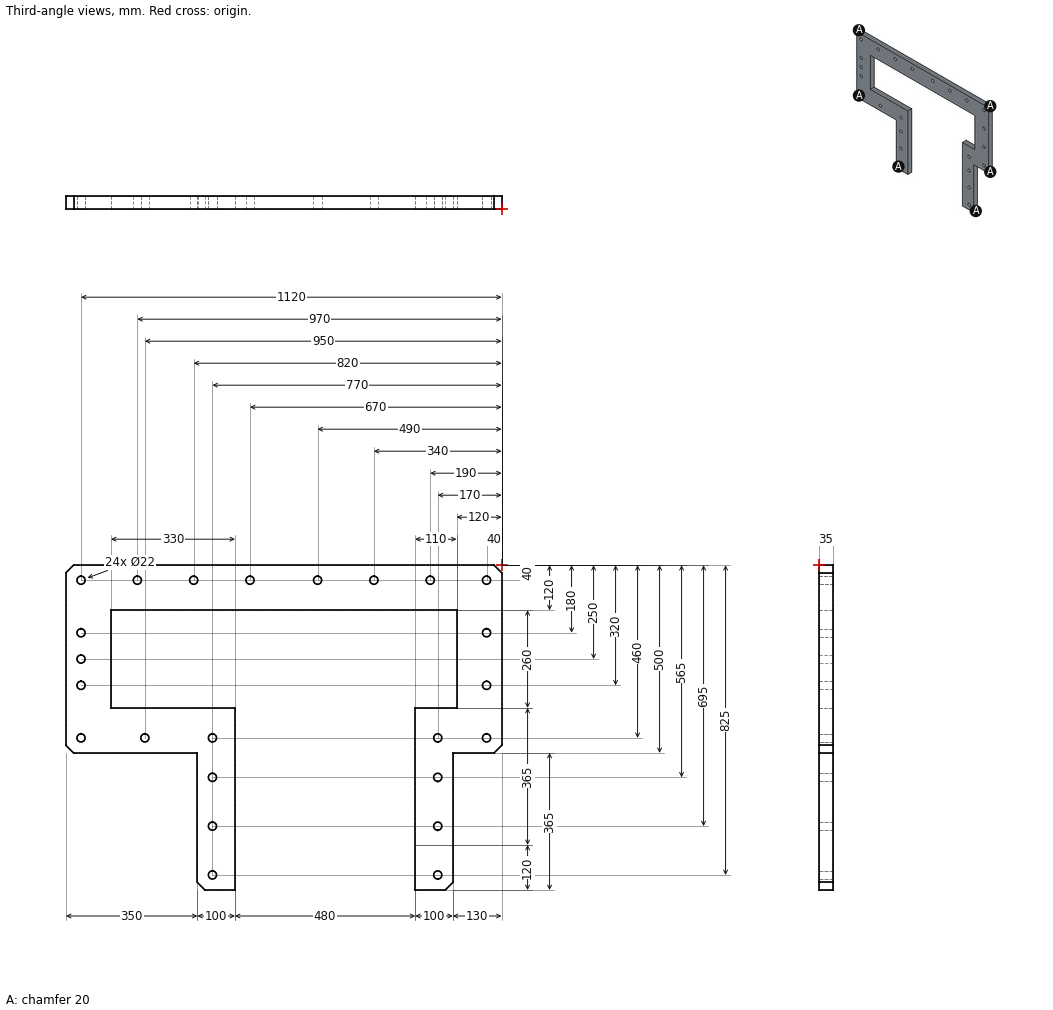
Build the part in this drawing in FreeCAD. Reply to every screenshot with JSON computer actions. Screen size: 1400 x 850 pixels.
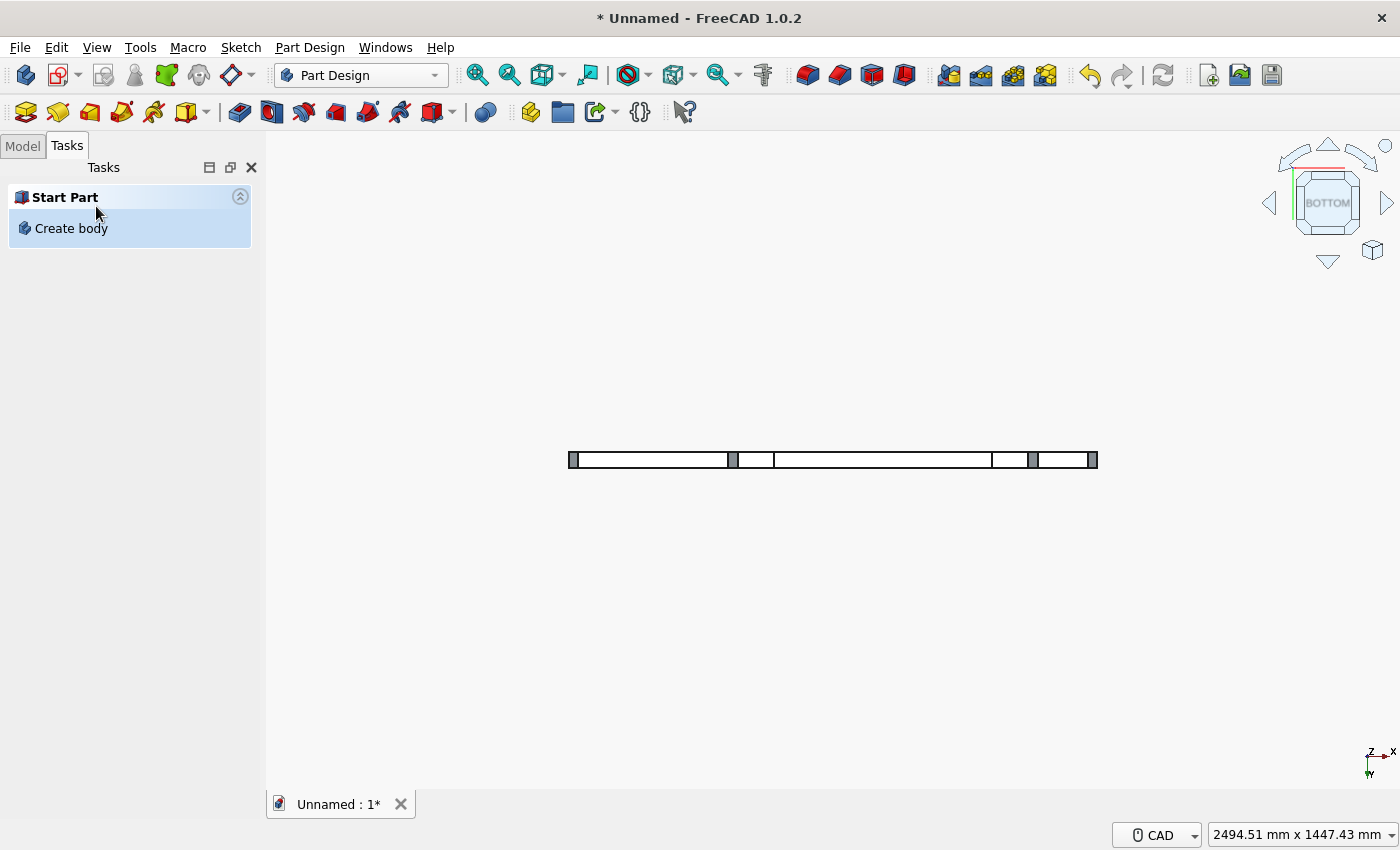
{"action": "key", "text": "4"}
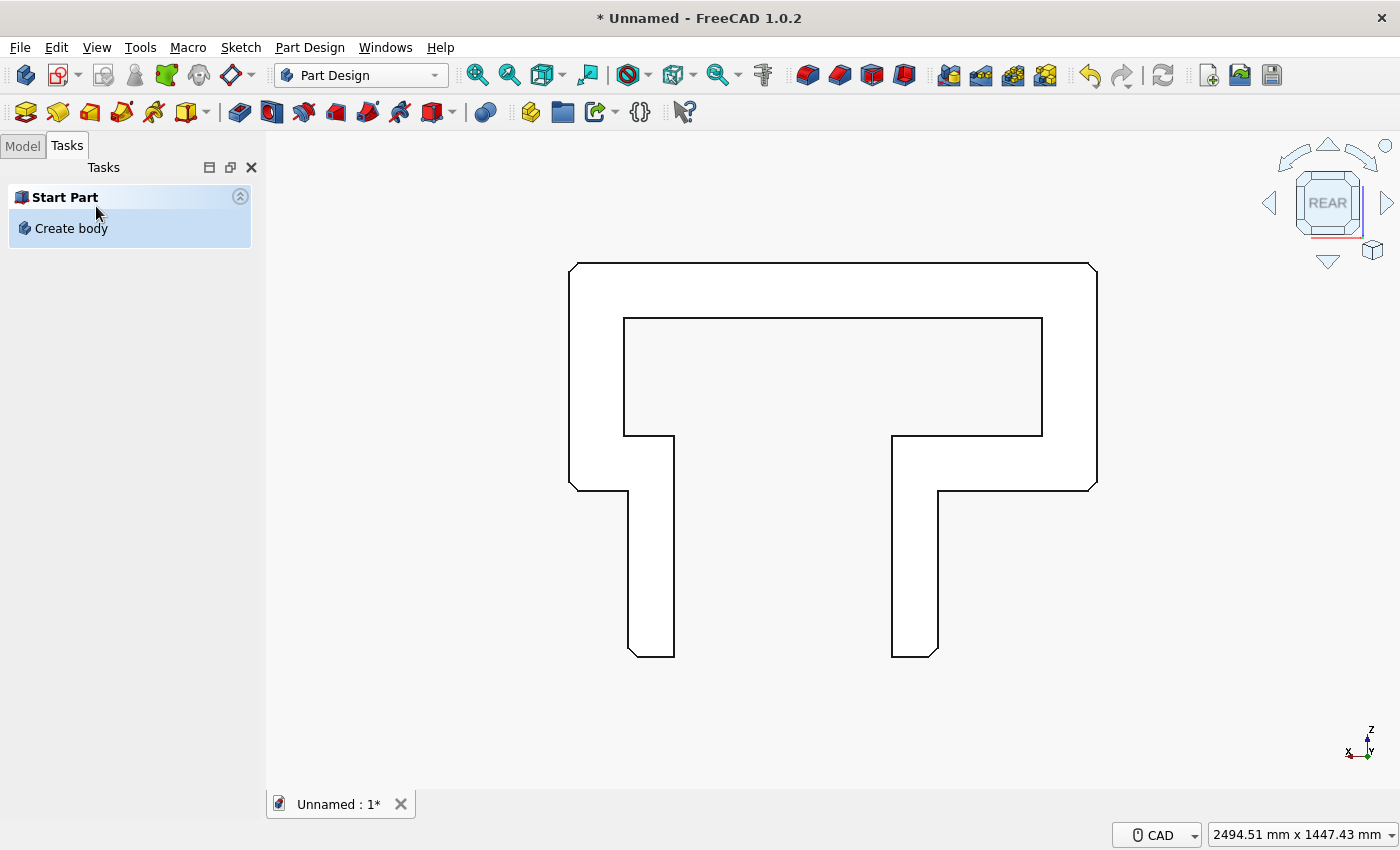
{"action": "left_click", "coordinate": [1059, 459]}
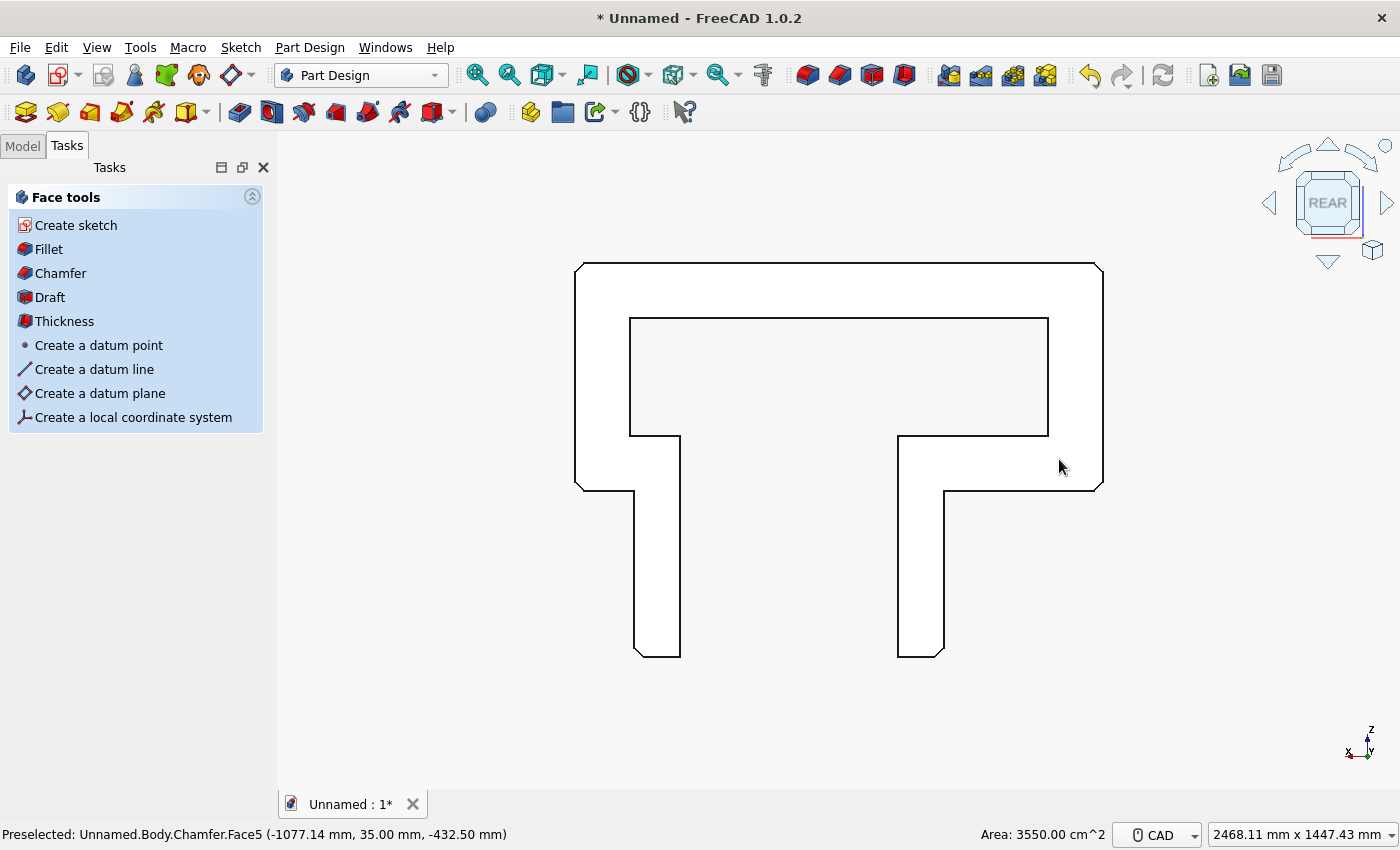
{"action": "left_click", "coordinate": [58, 76]}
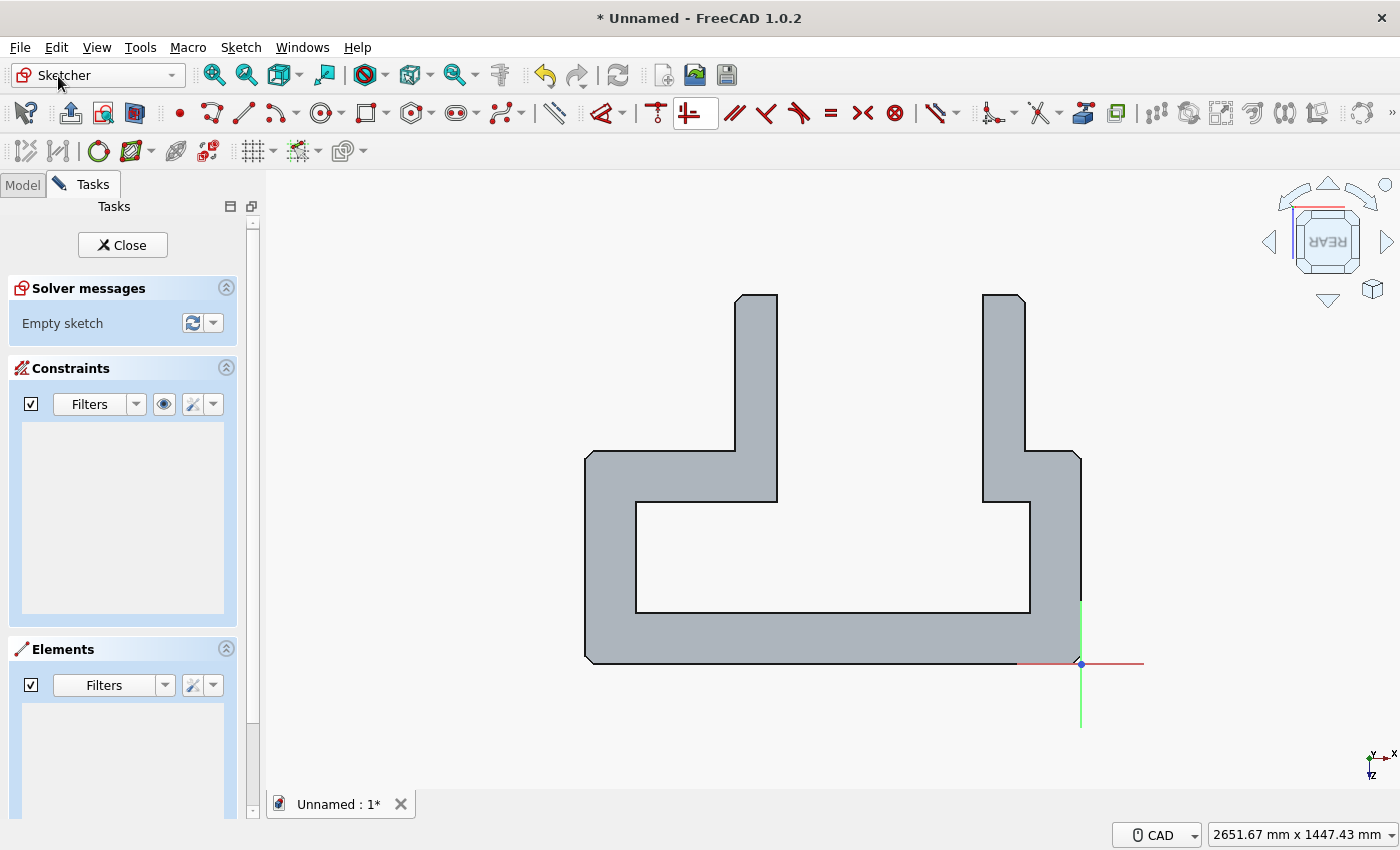
{"action": "key", "text": "g c"}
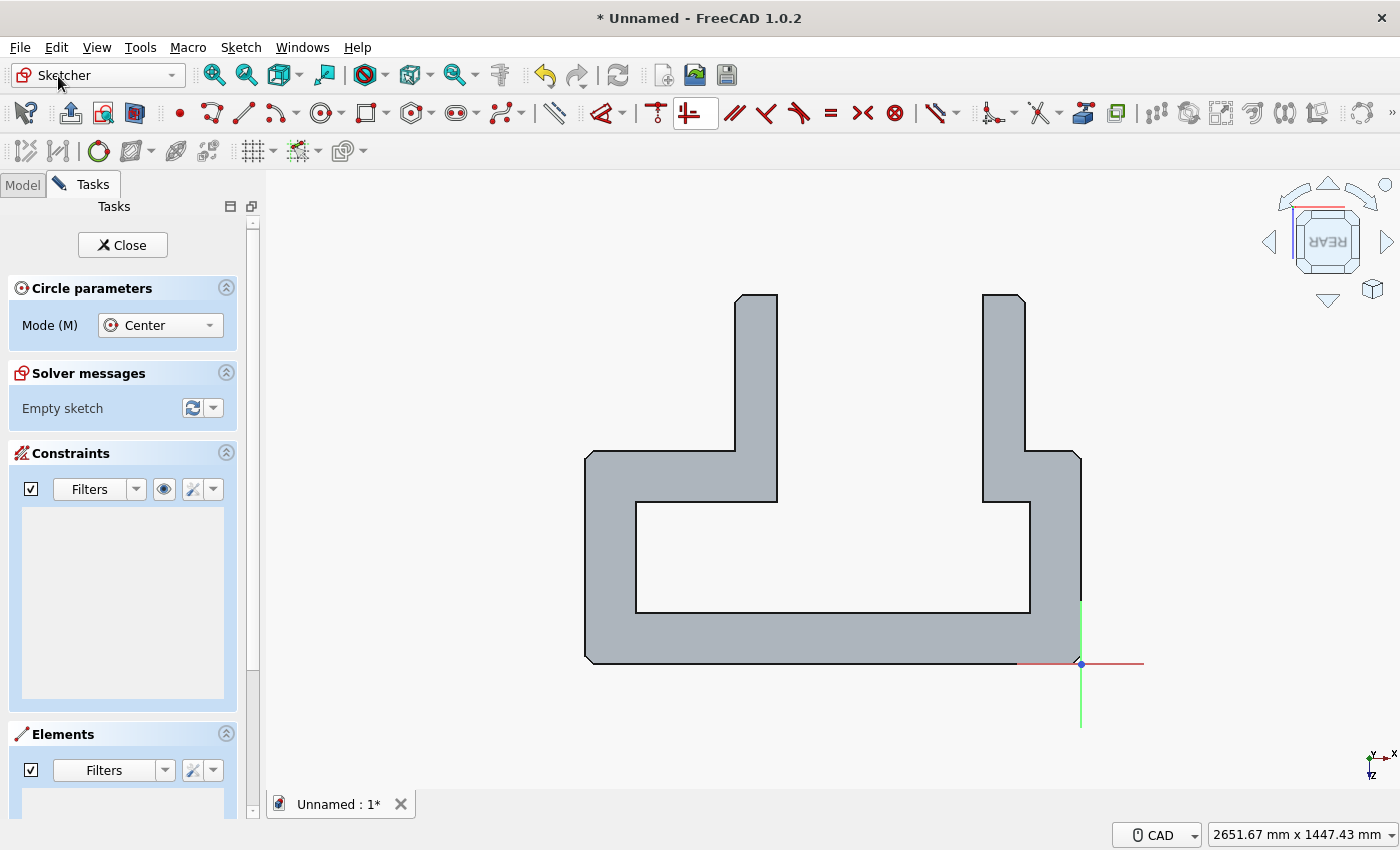
{"action": "scroll", "coordinate": [602, 647], "scroll_direction": "up", "scroll_amount": 8}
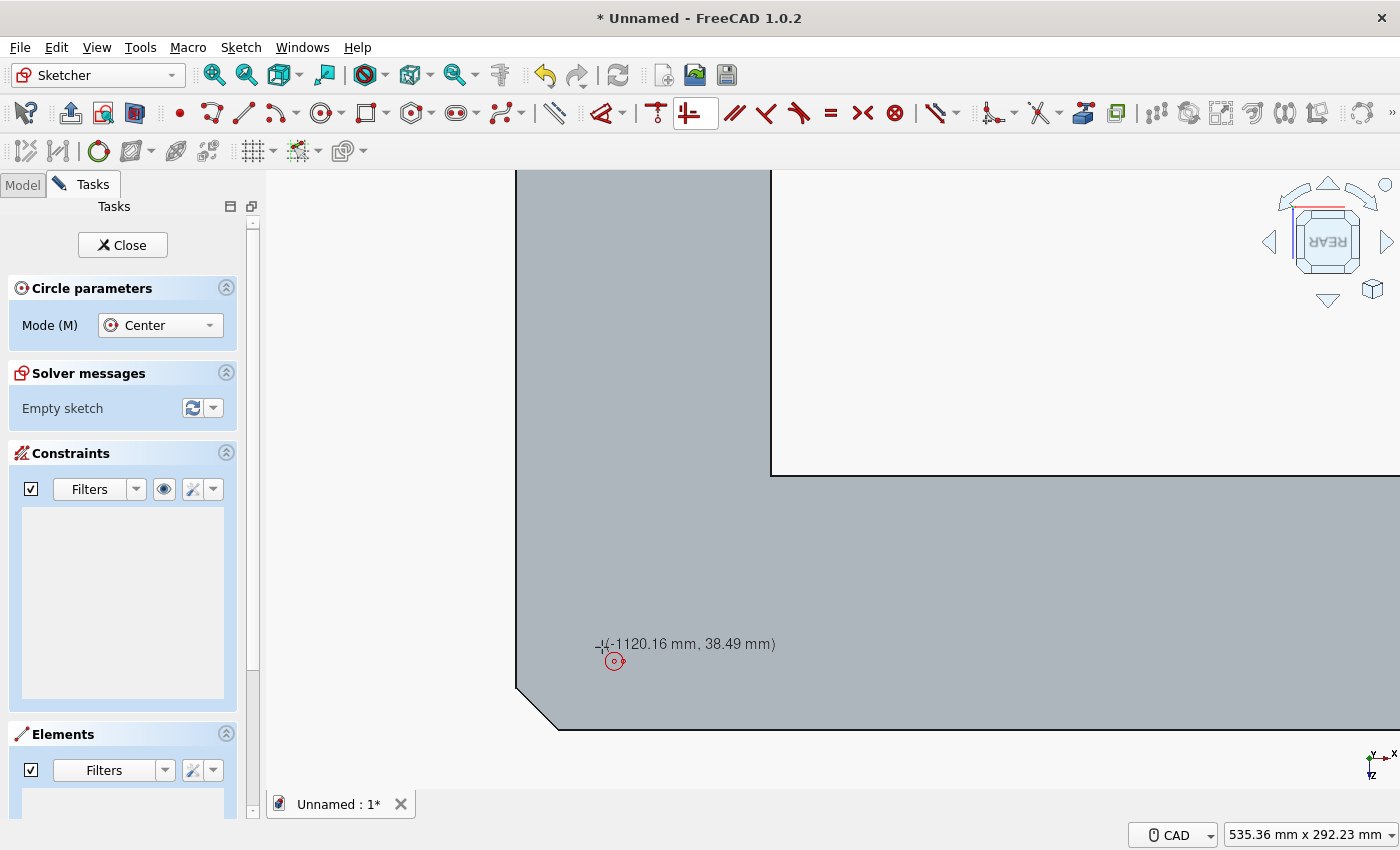
{"action": "scroll", "coordinate": [434, 687], "scroll_direction": "down", "scroll_amount": 7}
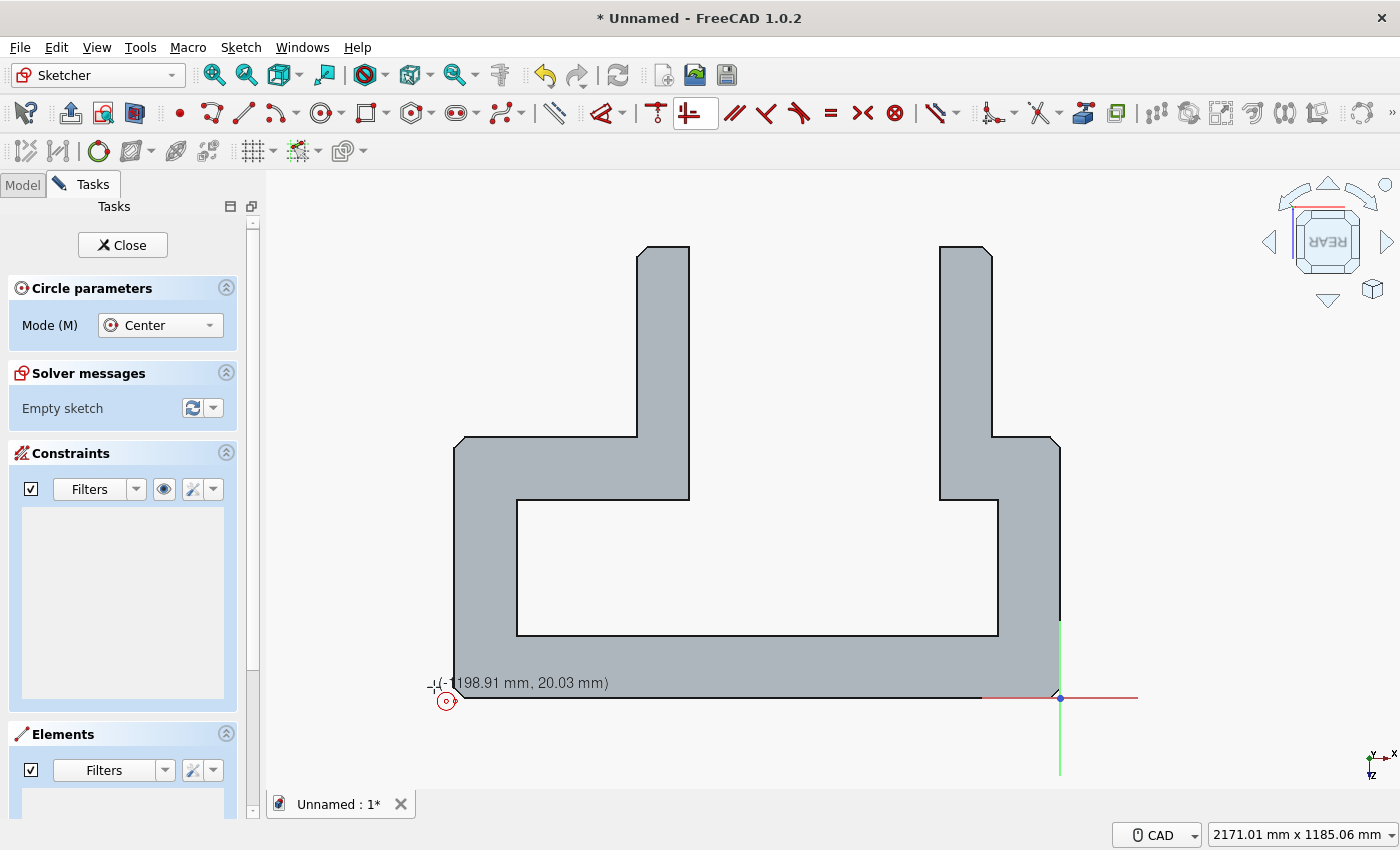
{"action": "left_click", "coordinate": [475, 677]}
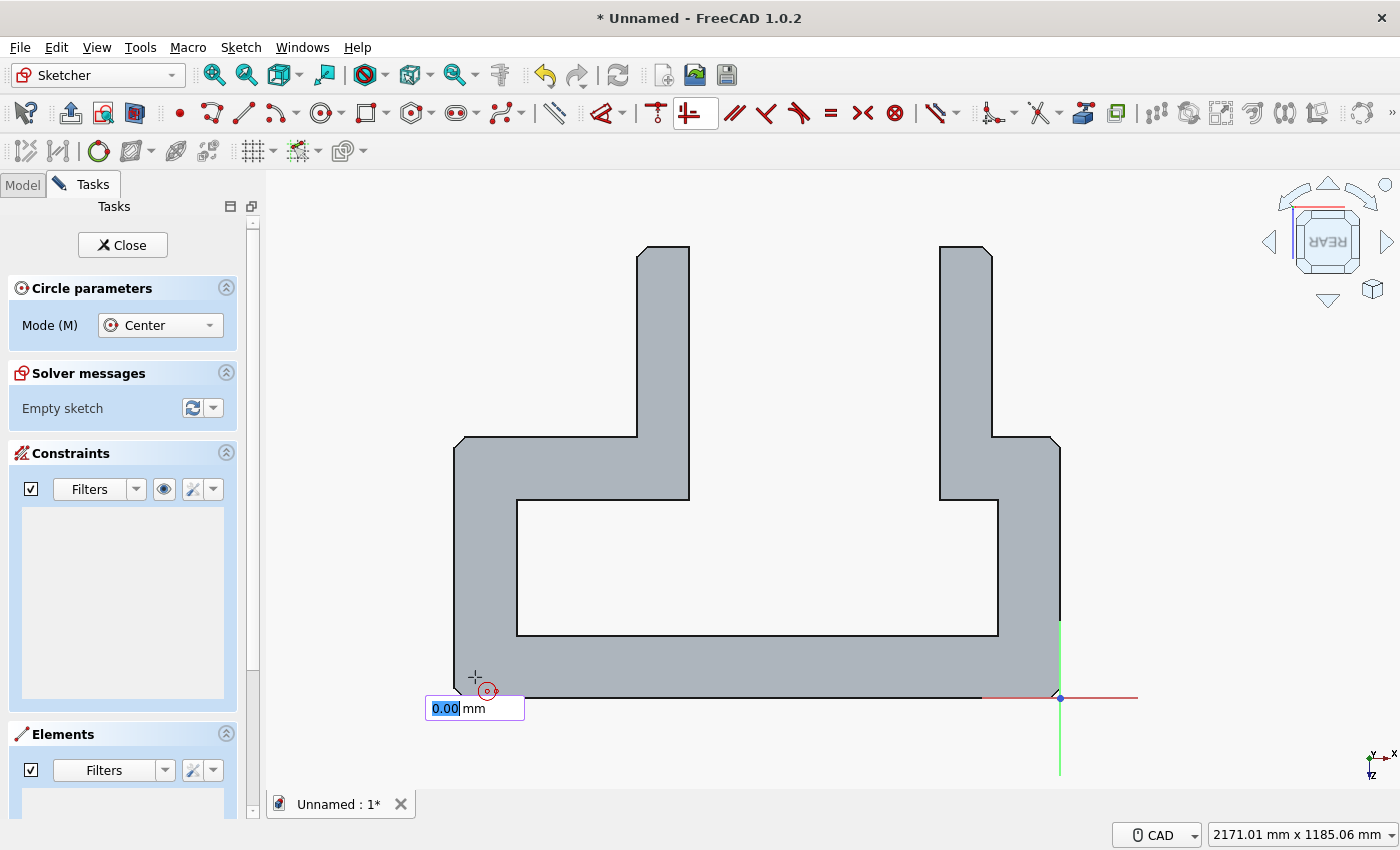
{"action": "scroll", "coordinate": [479, 673], "scroll_direction": "up", "scroll_amount": 6}